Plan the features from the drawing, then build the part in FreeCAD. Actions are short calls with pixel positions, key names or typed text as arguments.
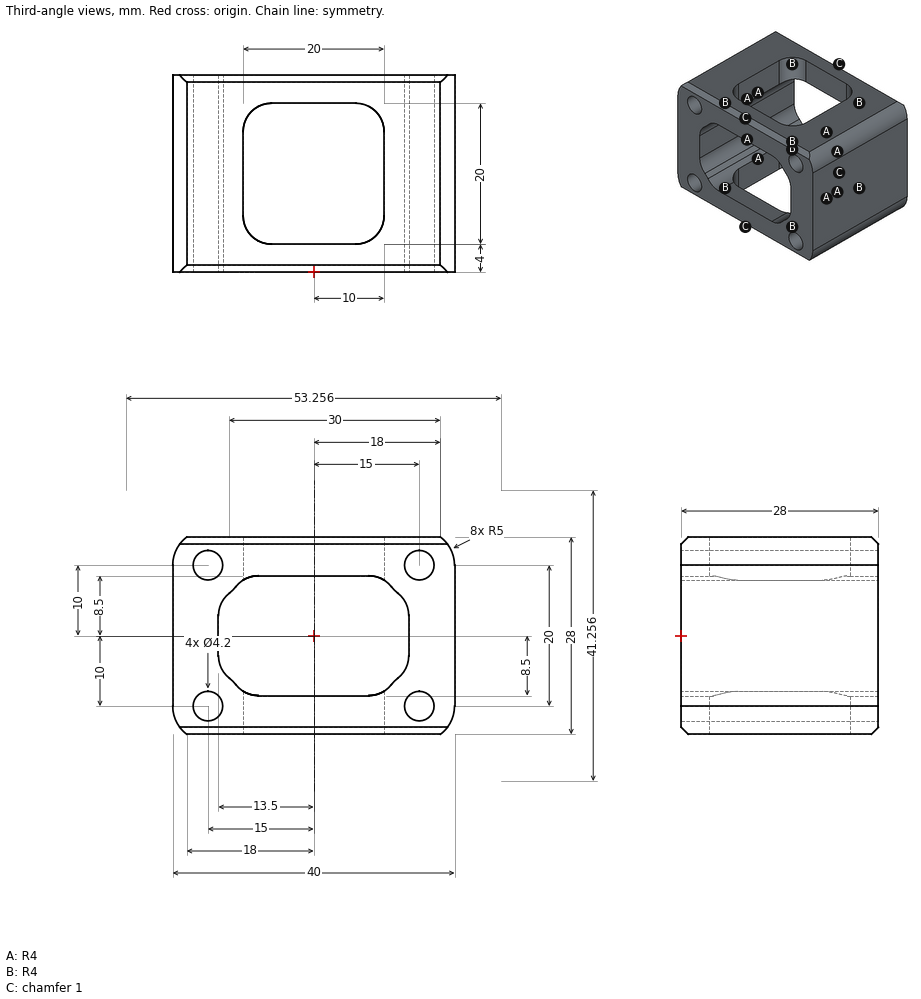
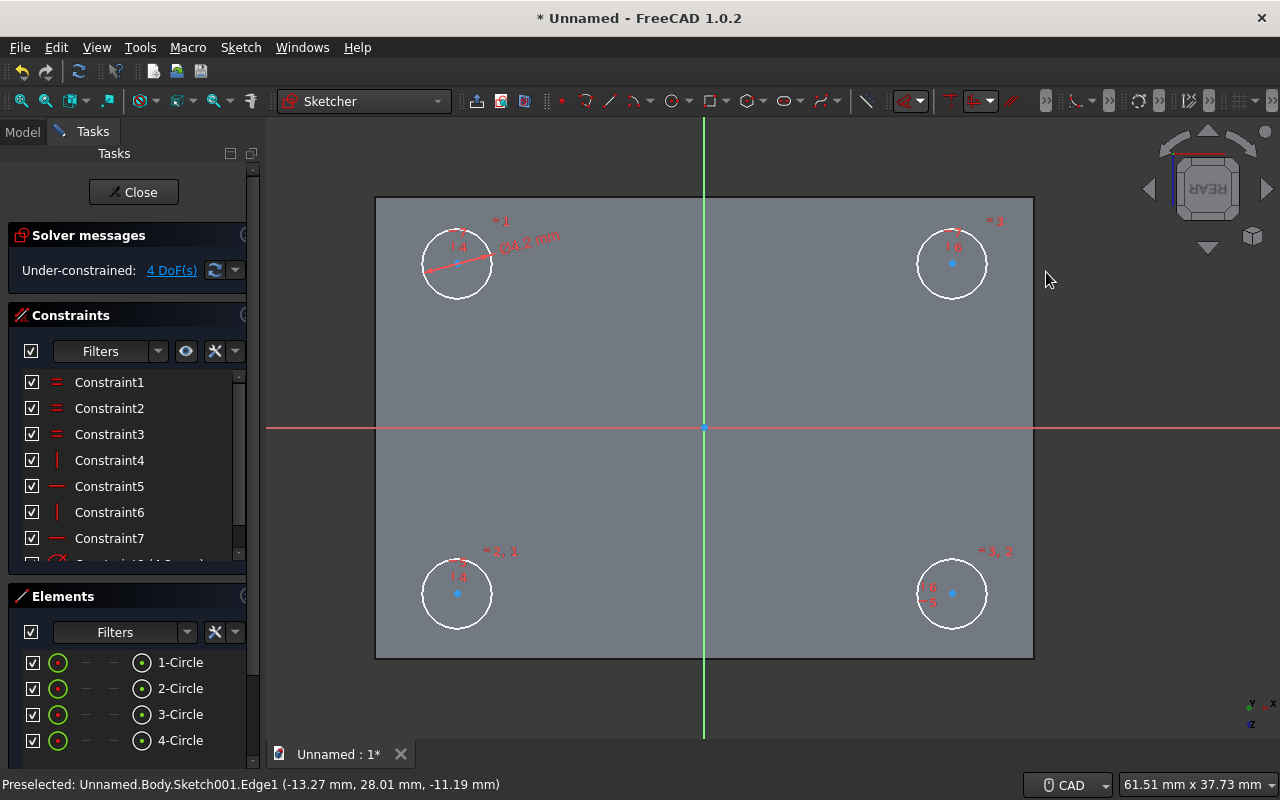
click(457, 264)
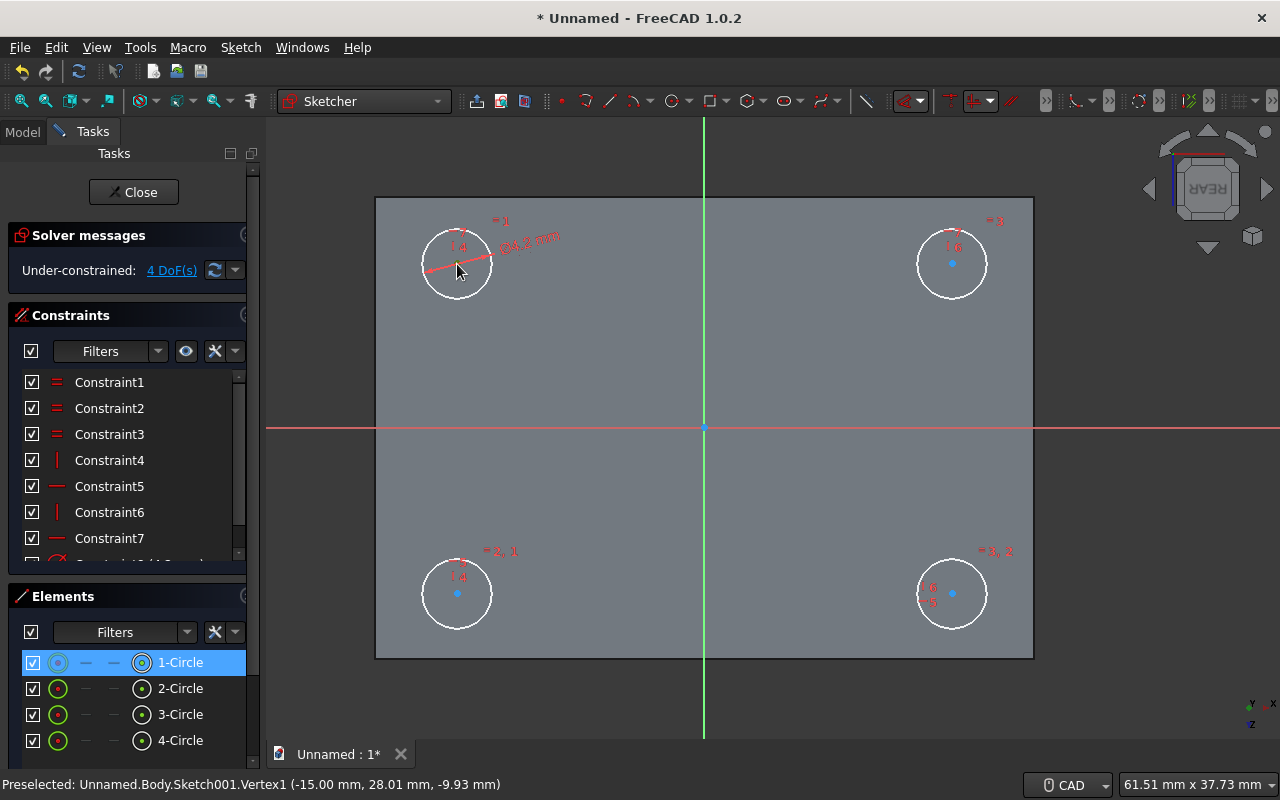
key(l)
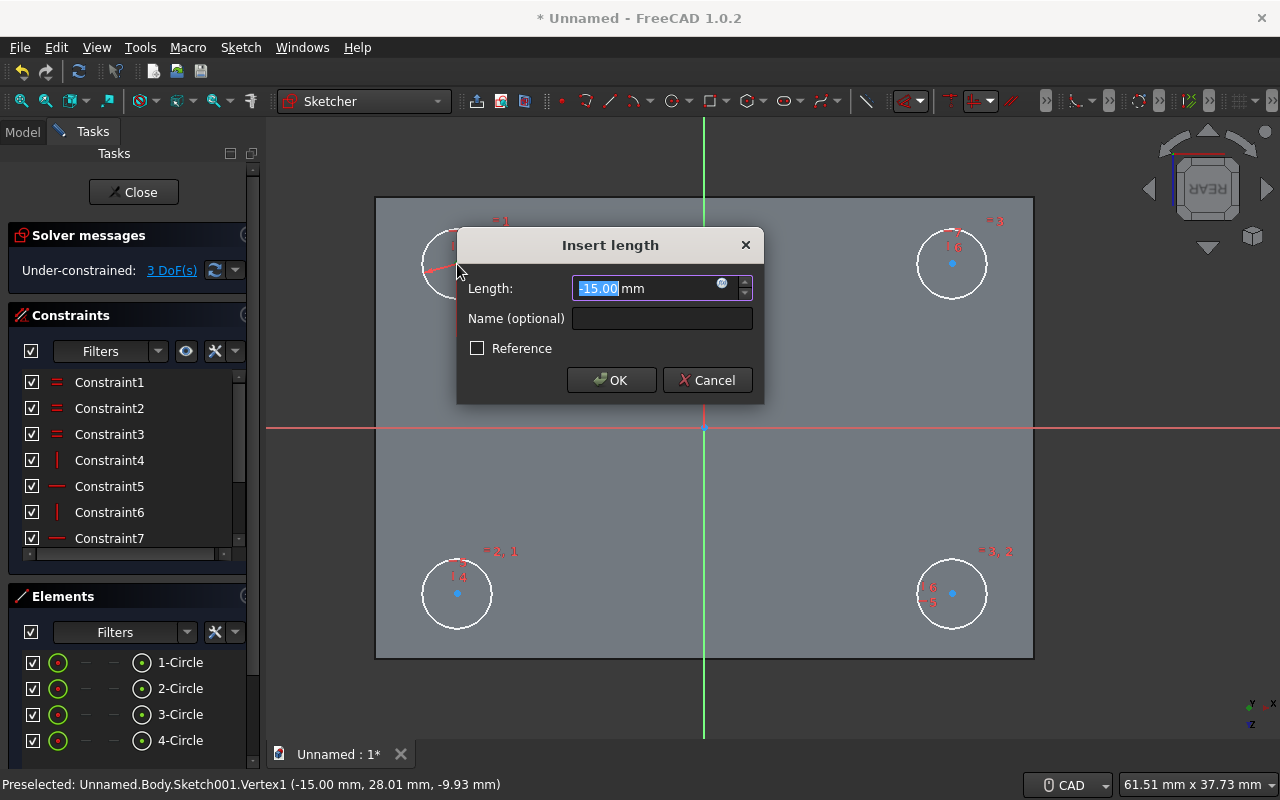
text(-15)
key(Return)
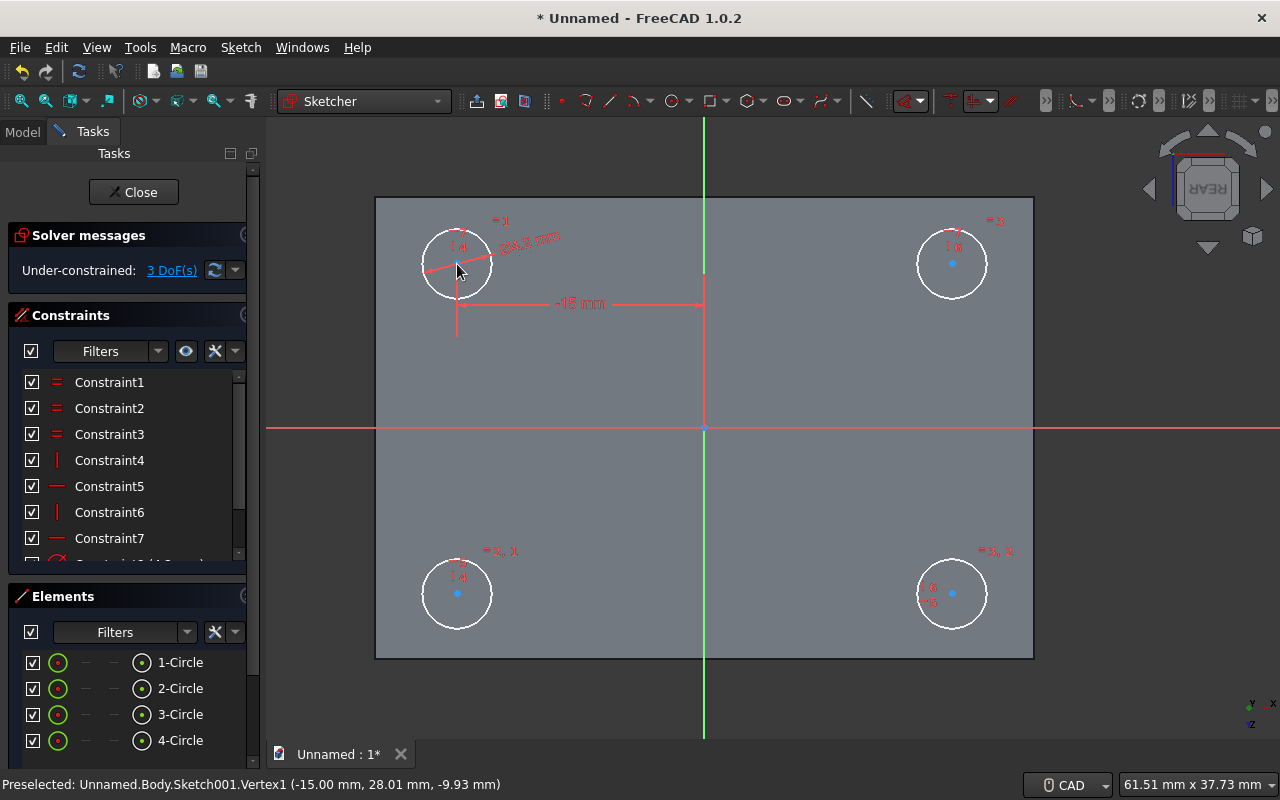
click(457, 264)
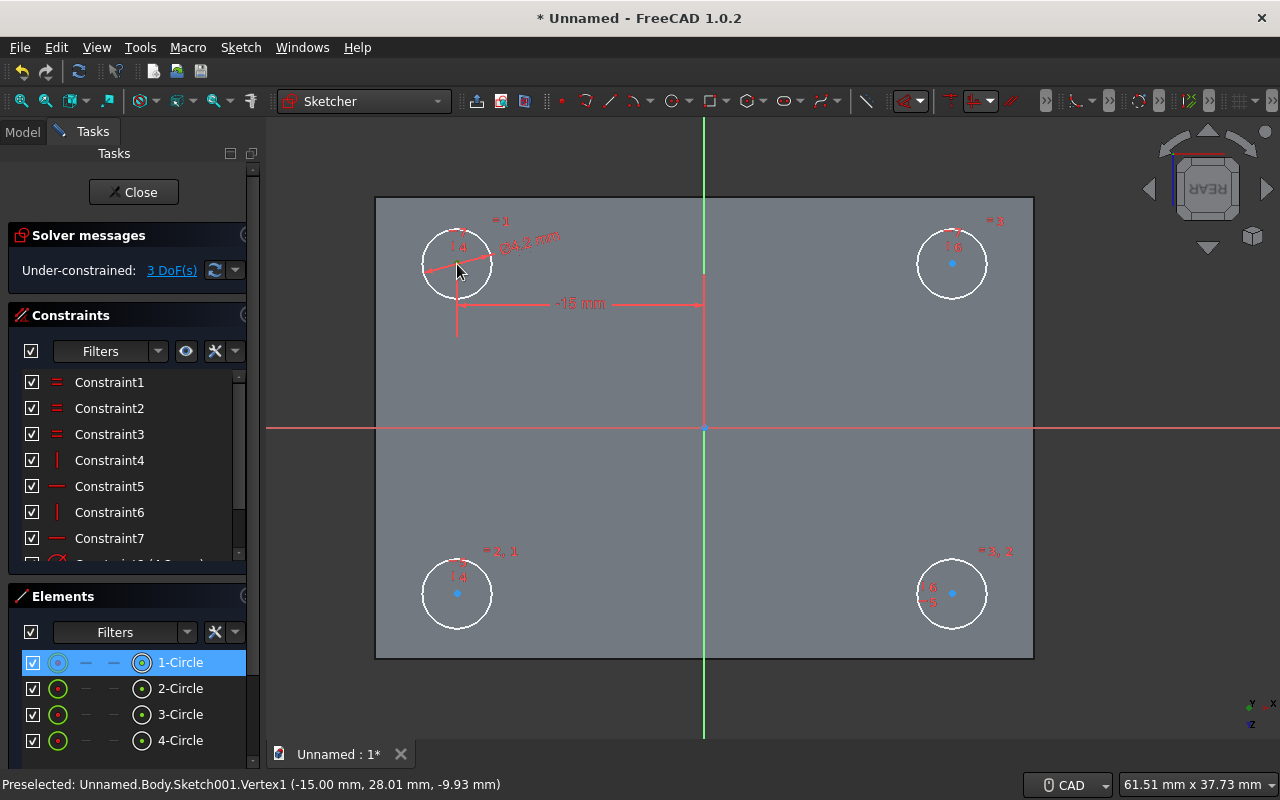
key(i)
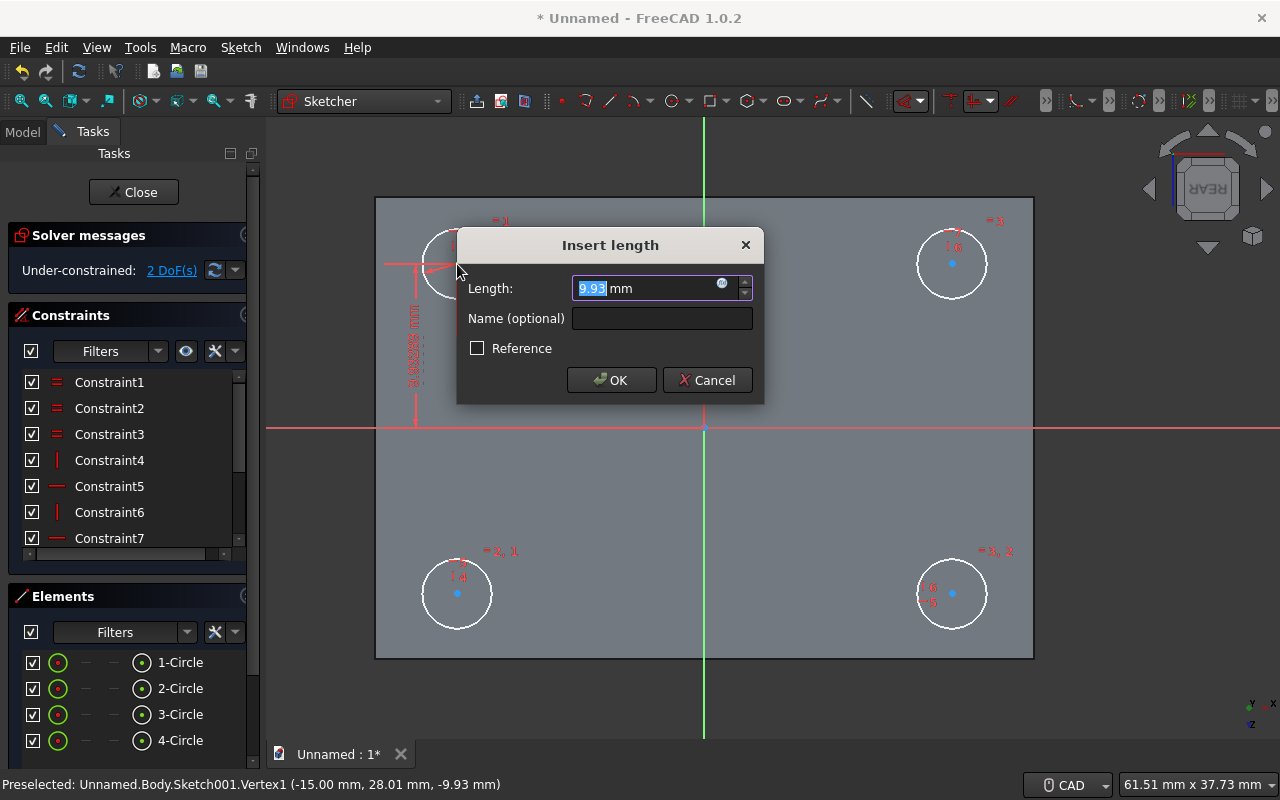
text(10)
key(Return)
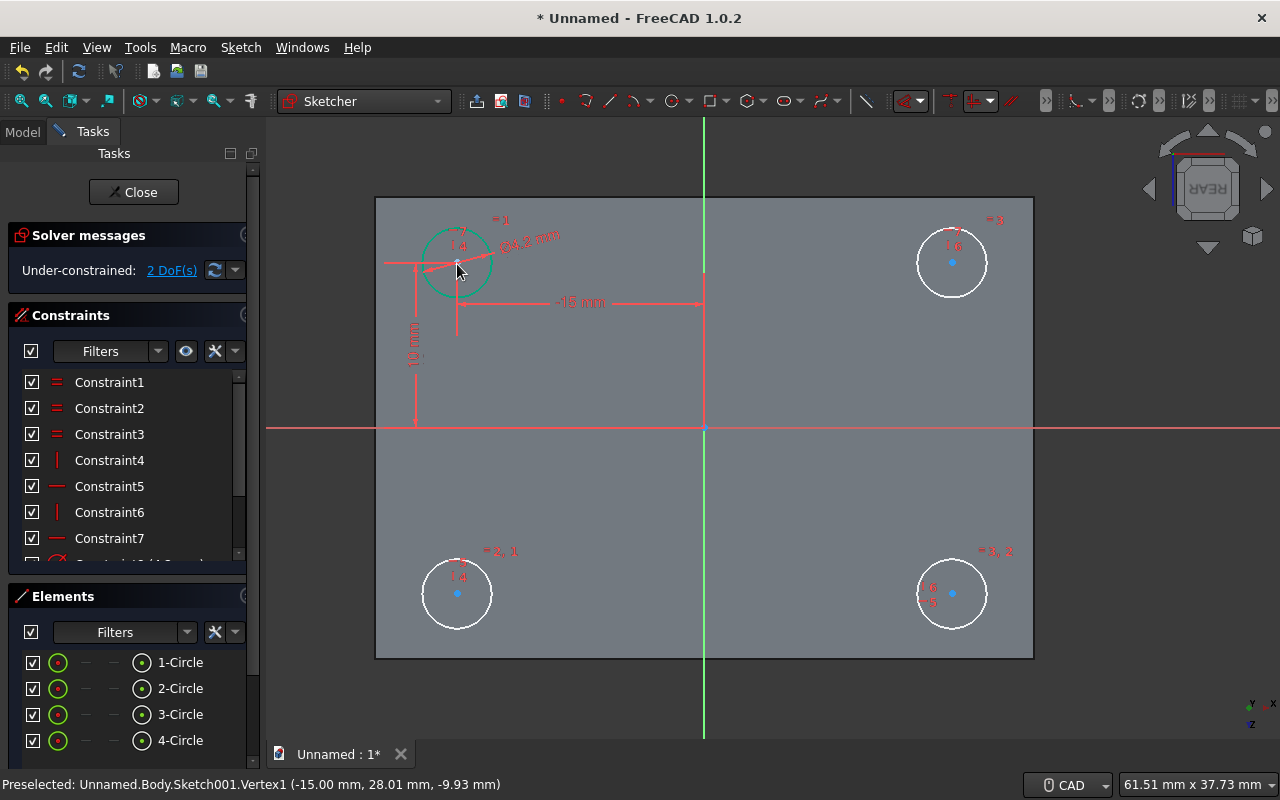
click(457, 594)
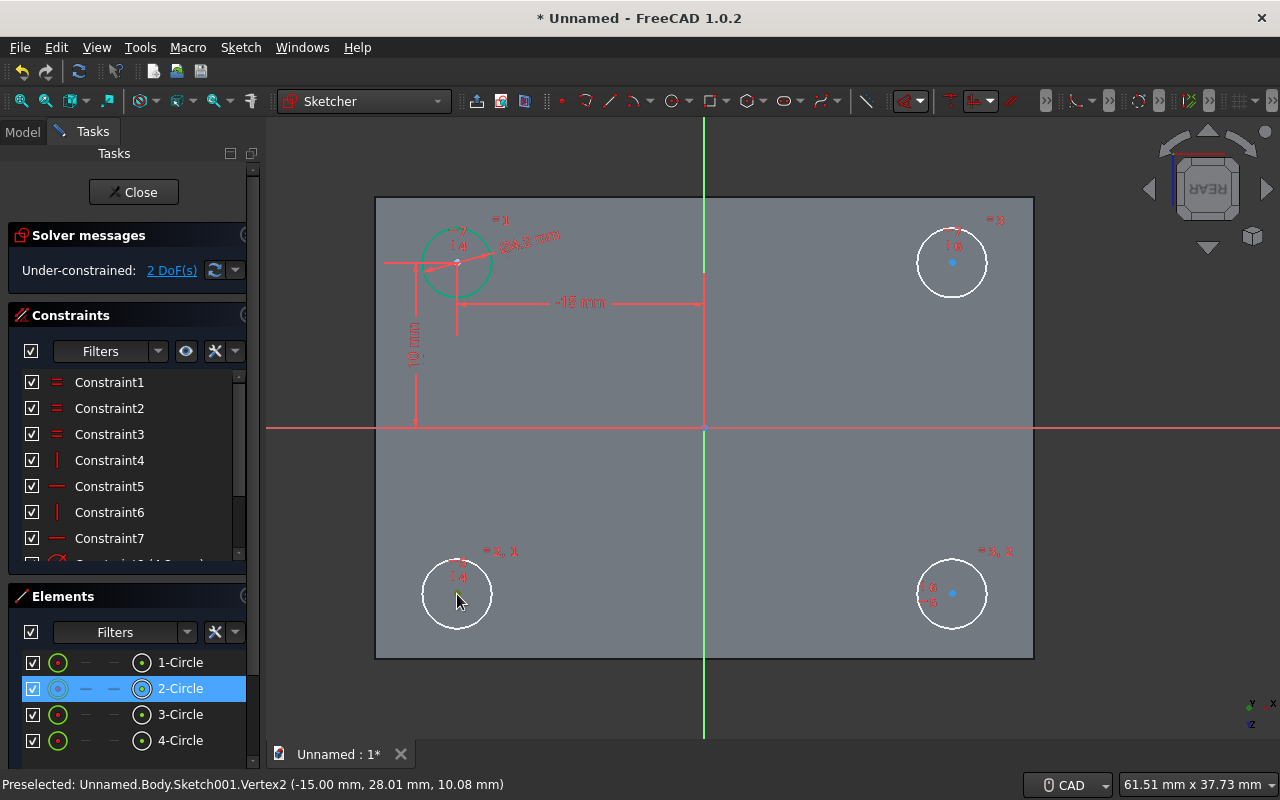
key(i)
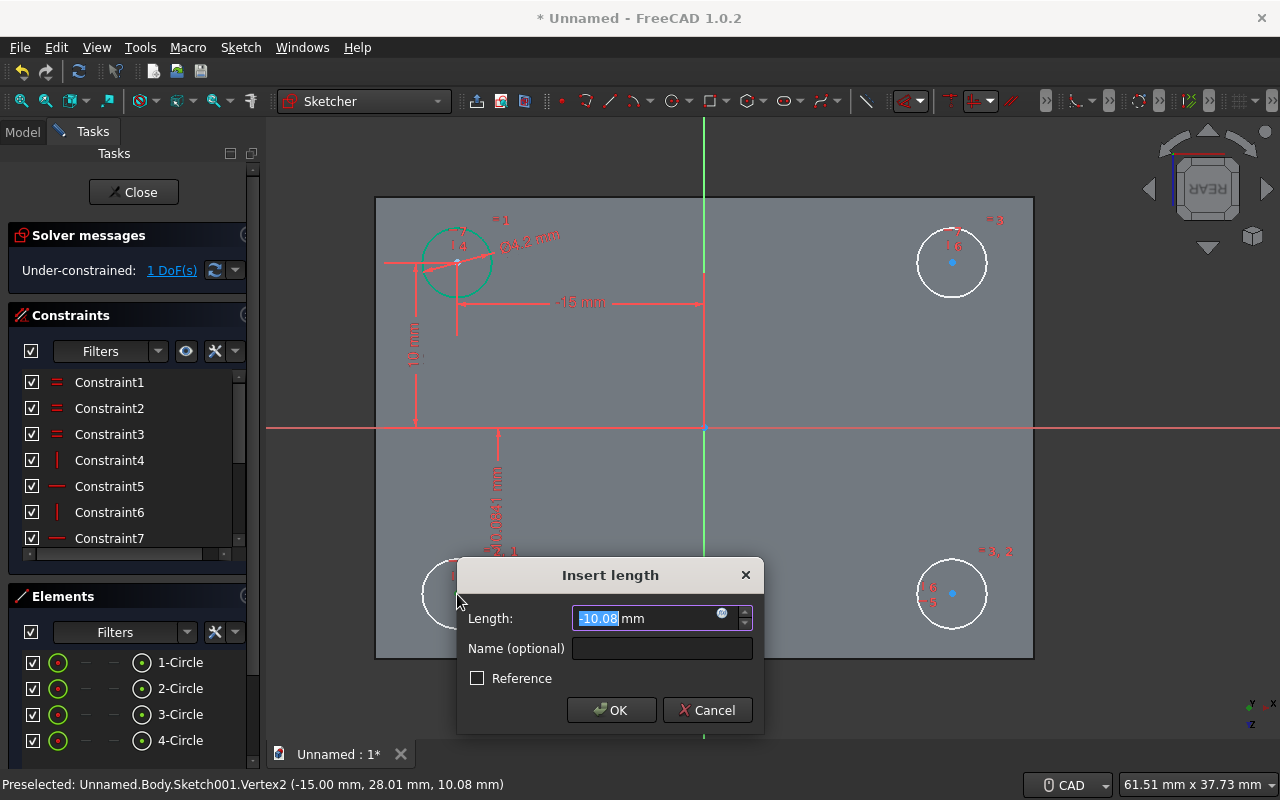
text(-10)
key(Return)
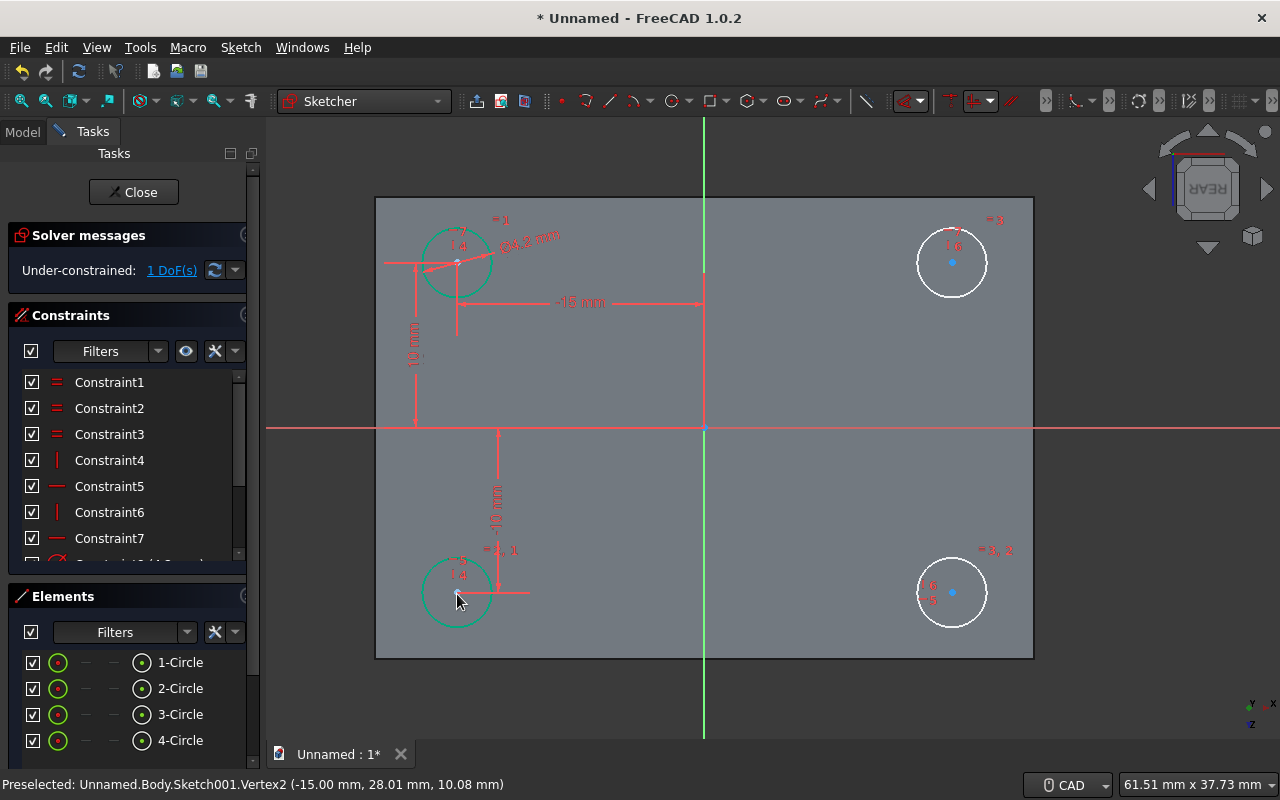
click(952, 593)